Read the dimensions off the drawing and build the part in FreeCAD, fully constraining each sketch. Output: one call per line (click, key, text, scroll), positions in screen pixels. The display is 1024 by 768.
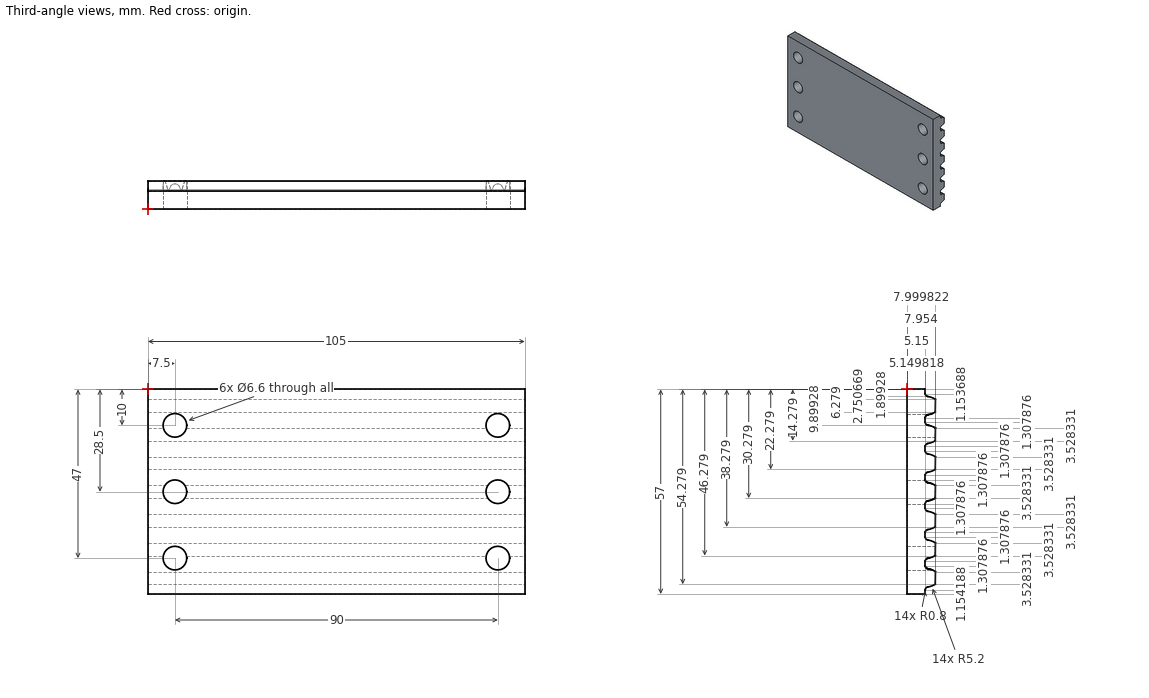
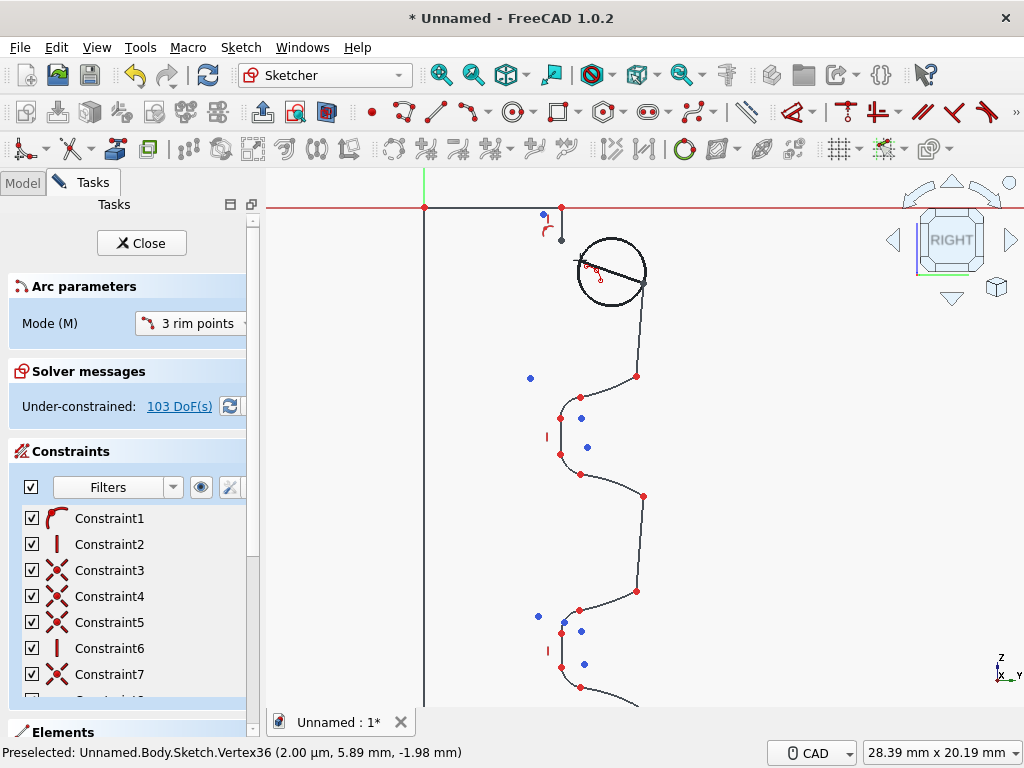
scroll(610, 267, up, 8)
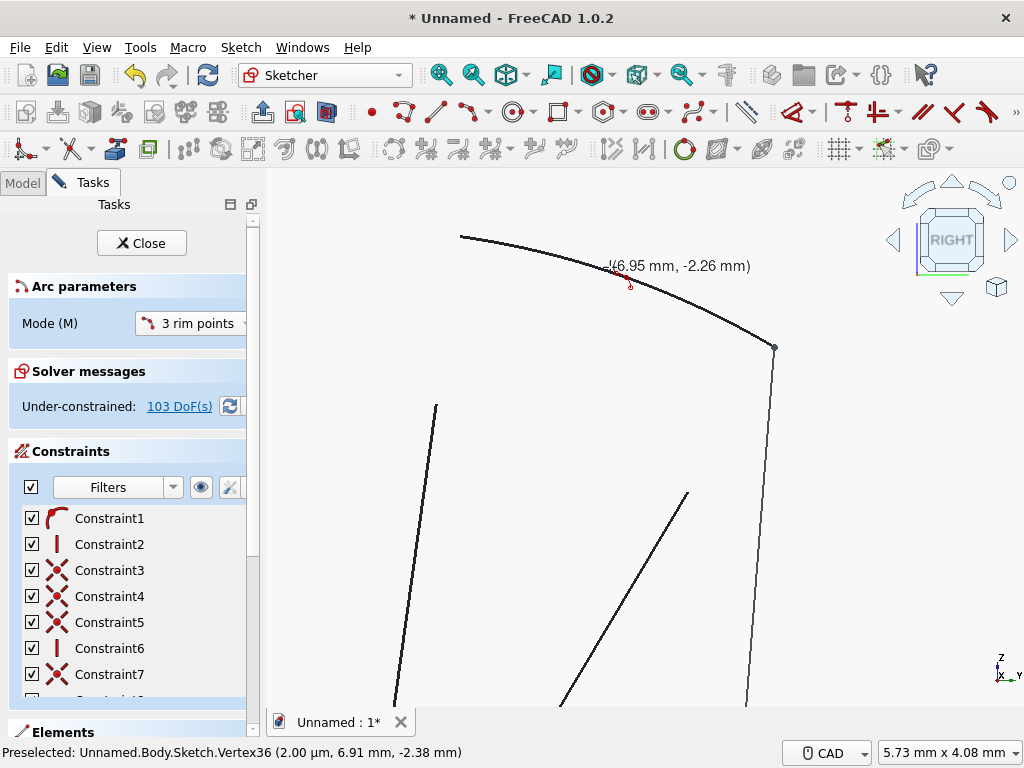
click(610, 267)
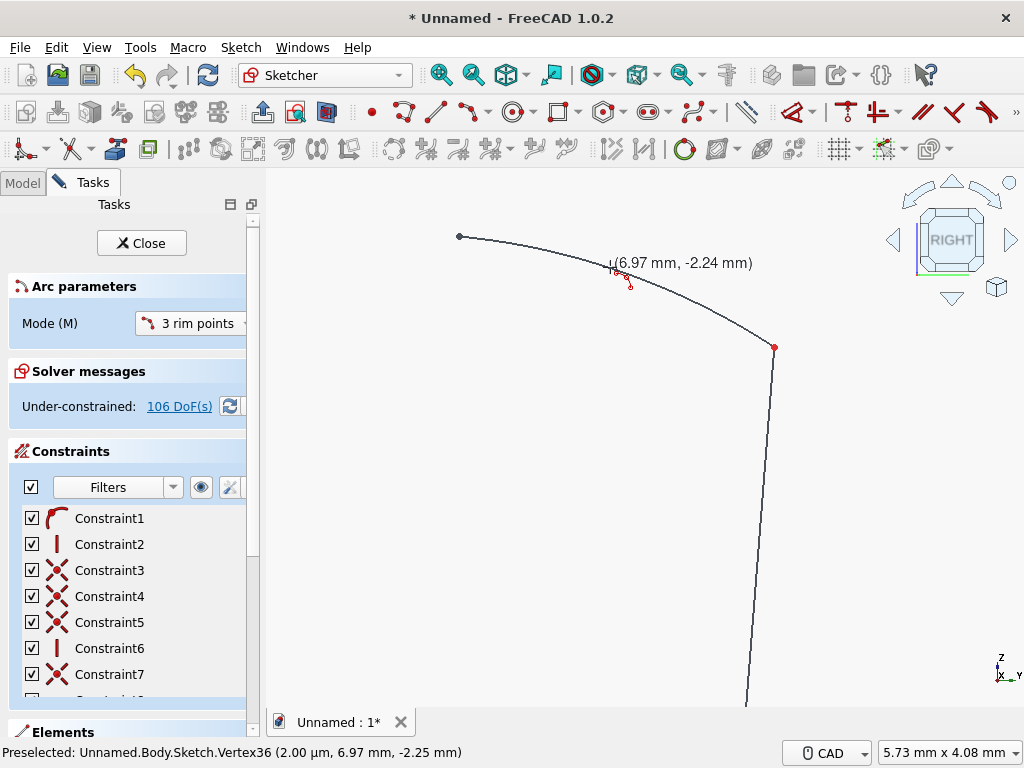
scroll(595, 264, down, 15)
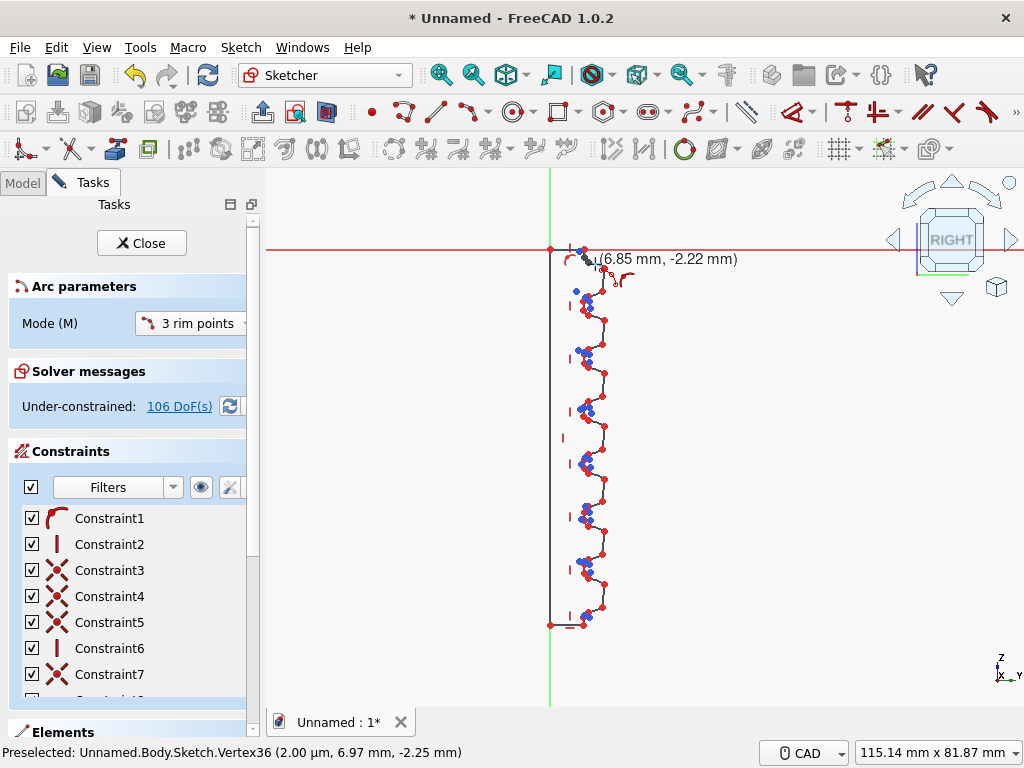
scroll(589, 262, up, 7)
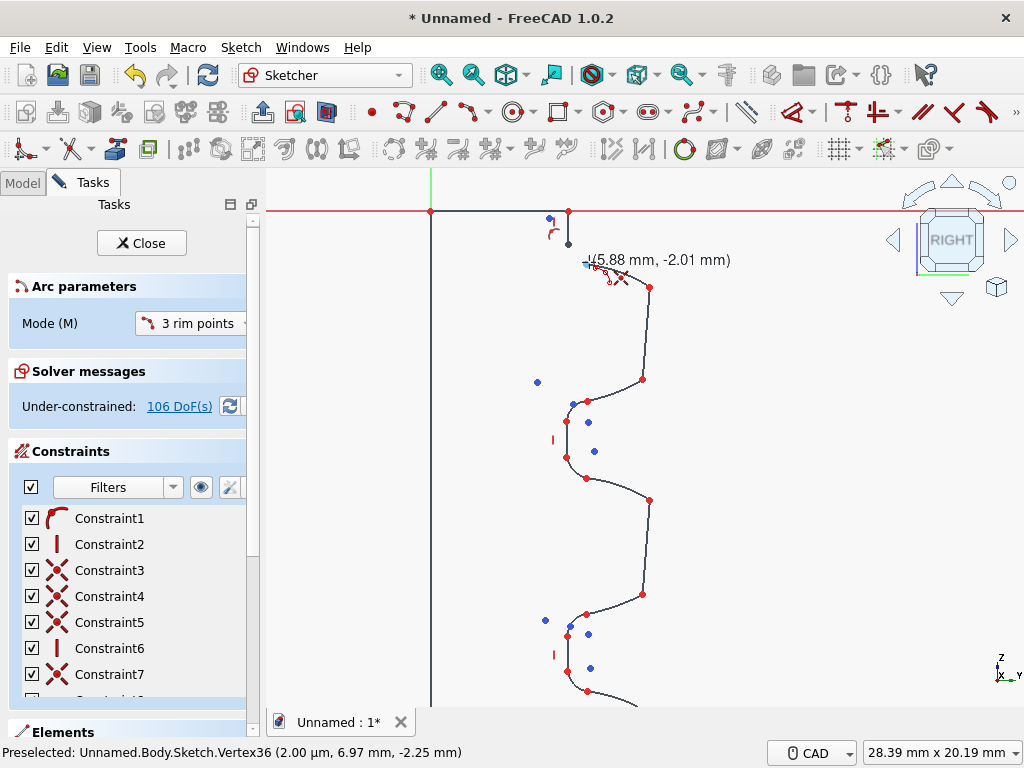
click(586, 265)
click(568, 244)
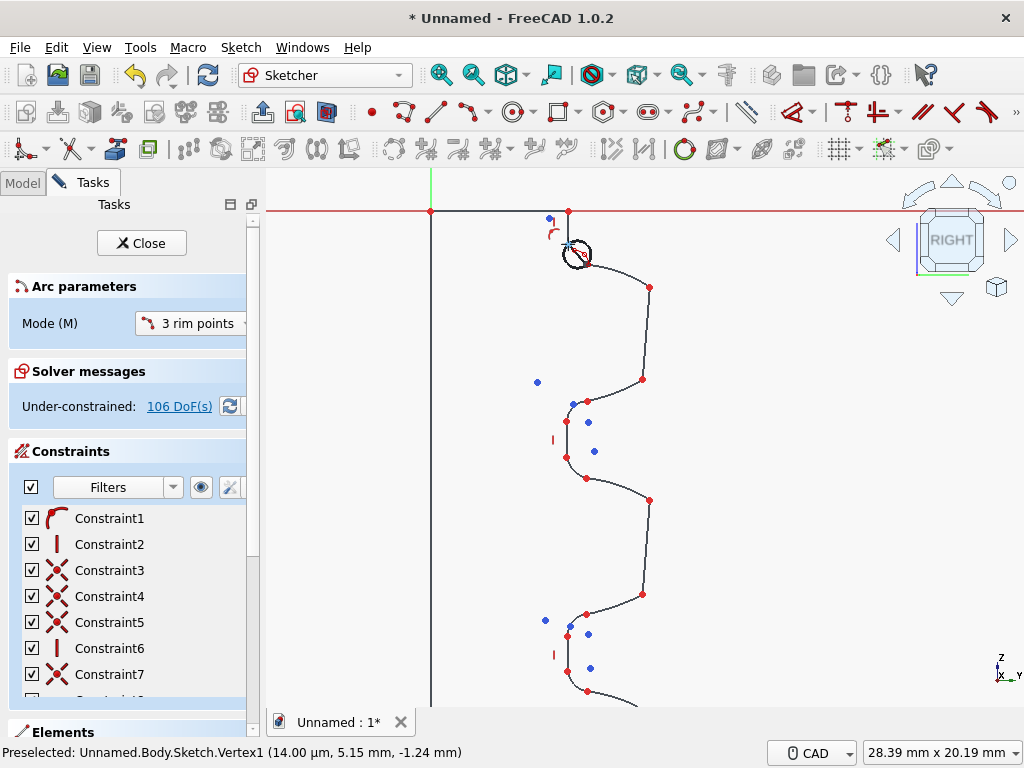
scroll(573, 256, up, 6)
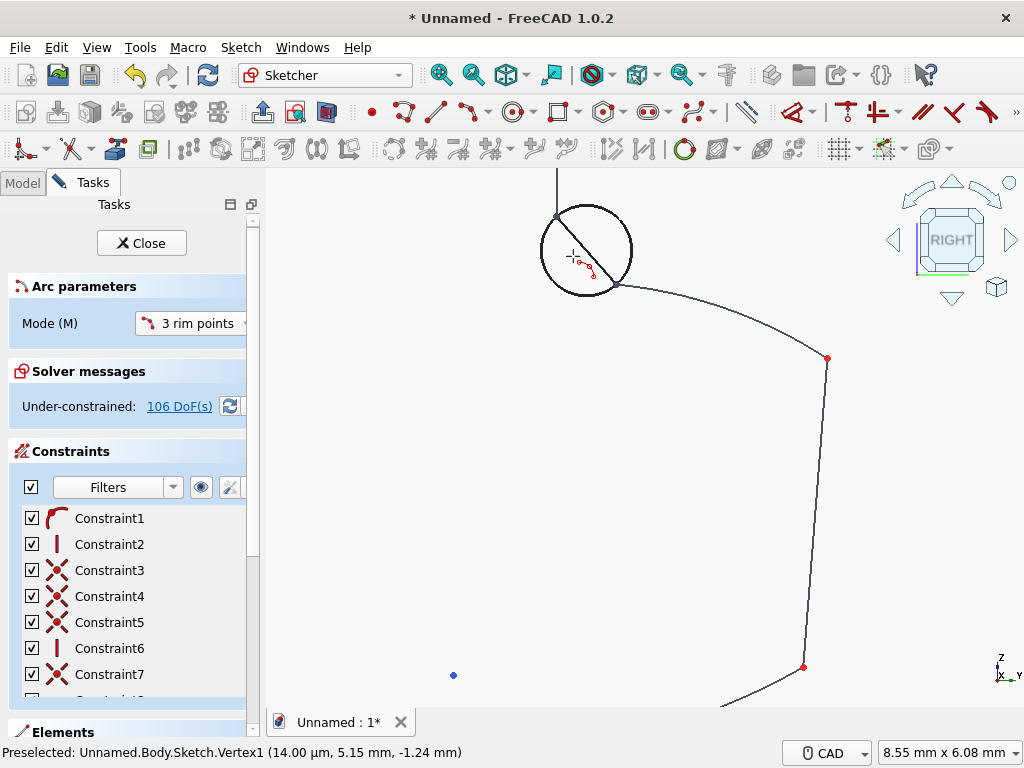
click(574, 256)
key(Escape)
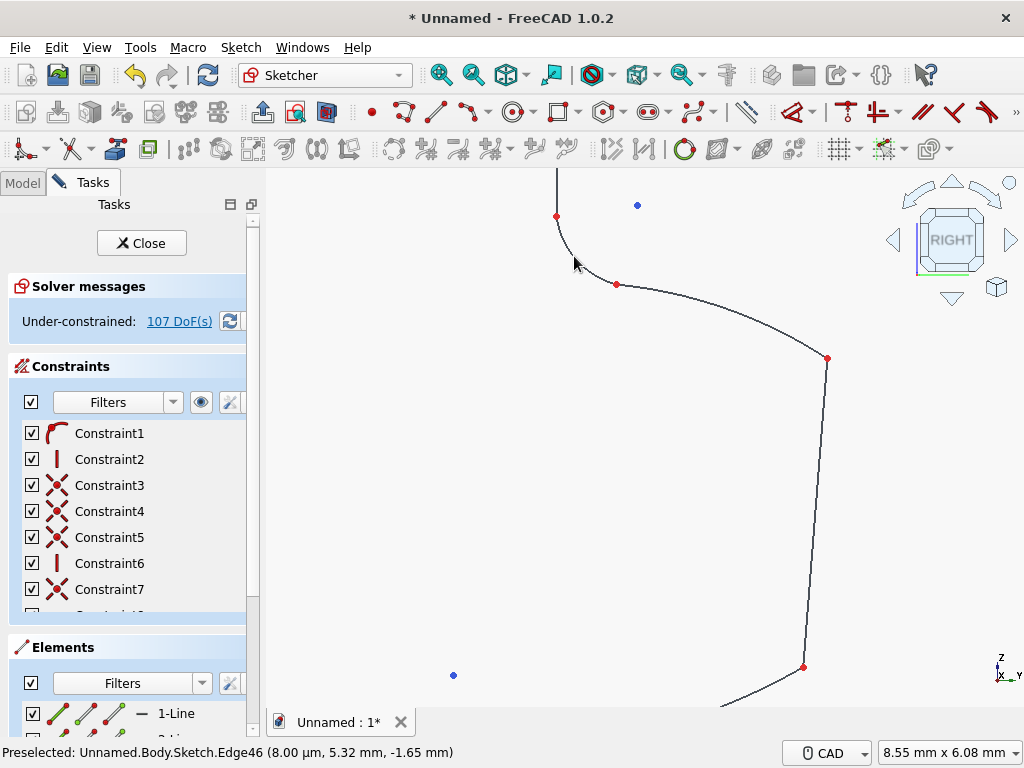
scroll(586, 261, down, 13)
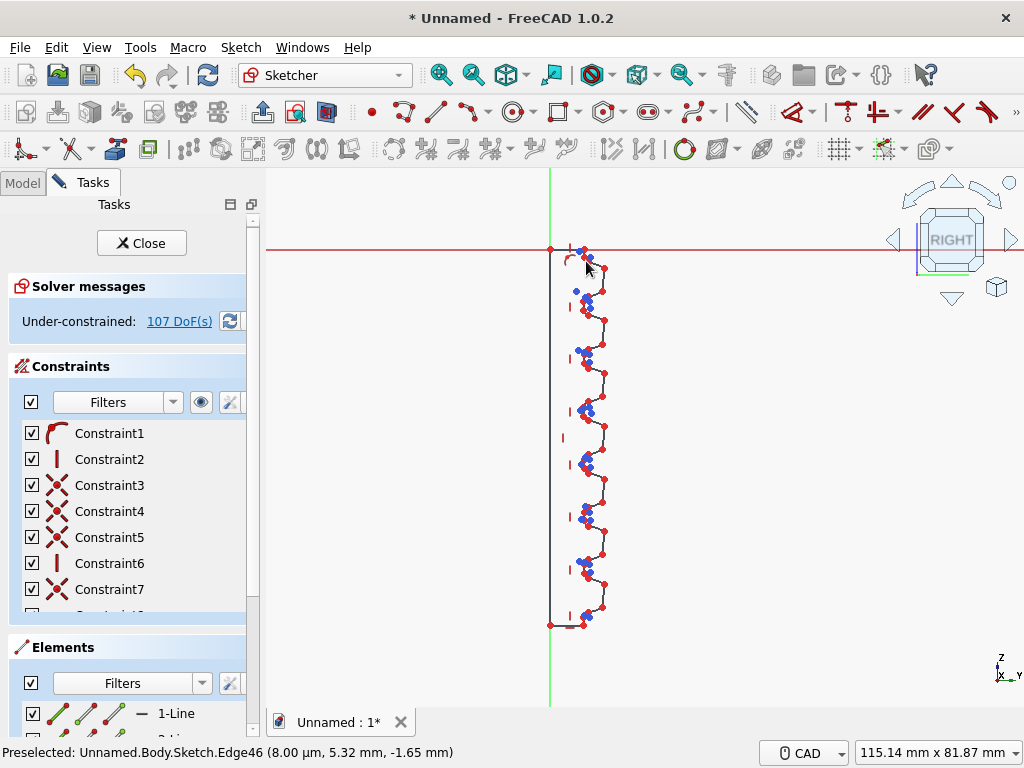
scroll(584, 255, up, 9)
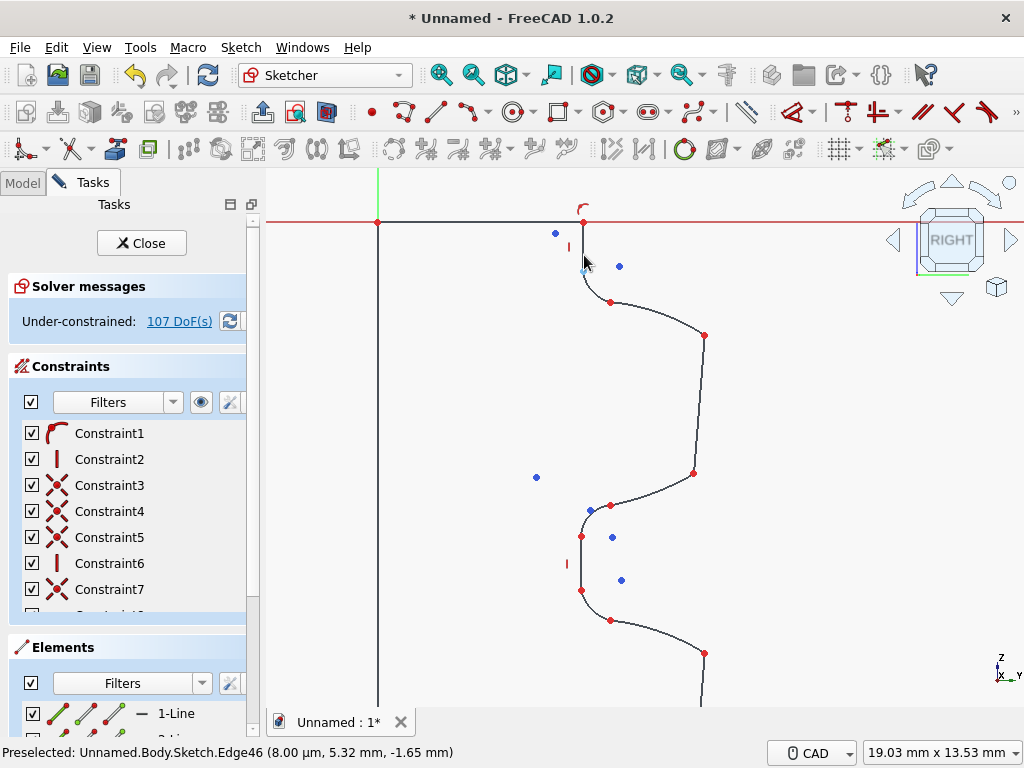
click(583, 257)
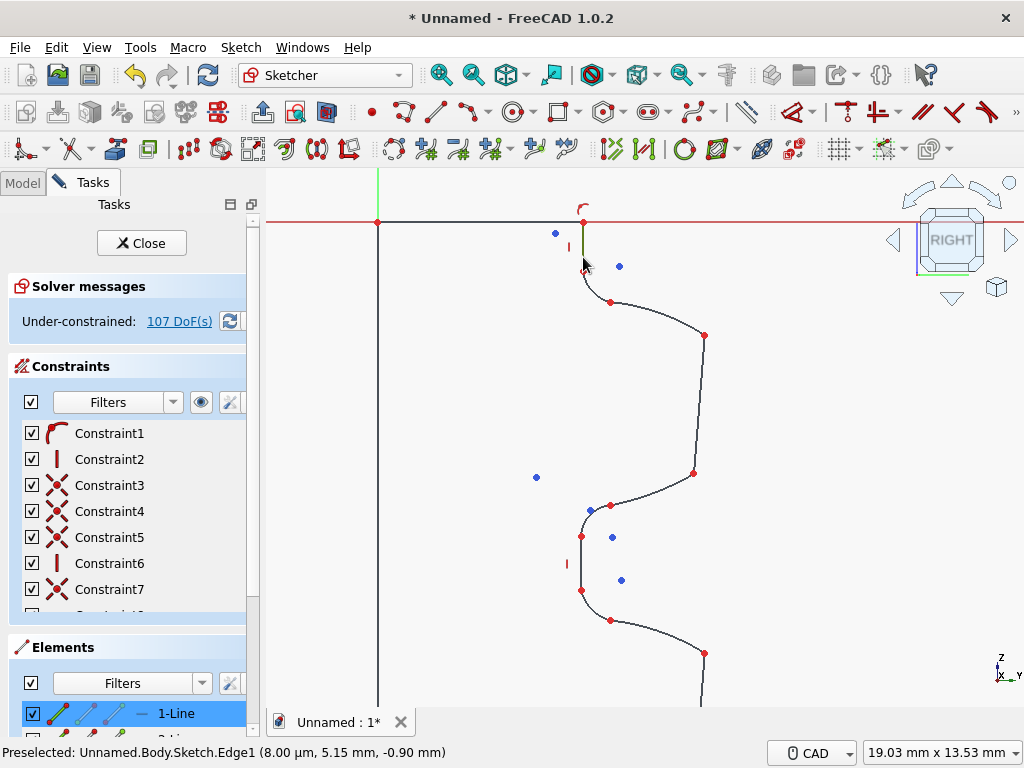
click(587, 284)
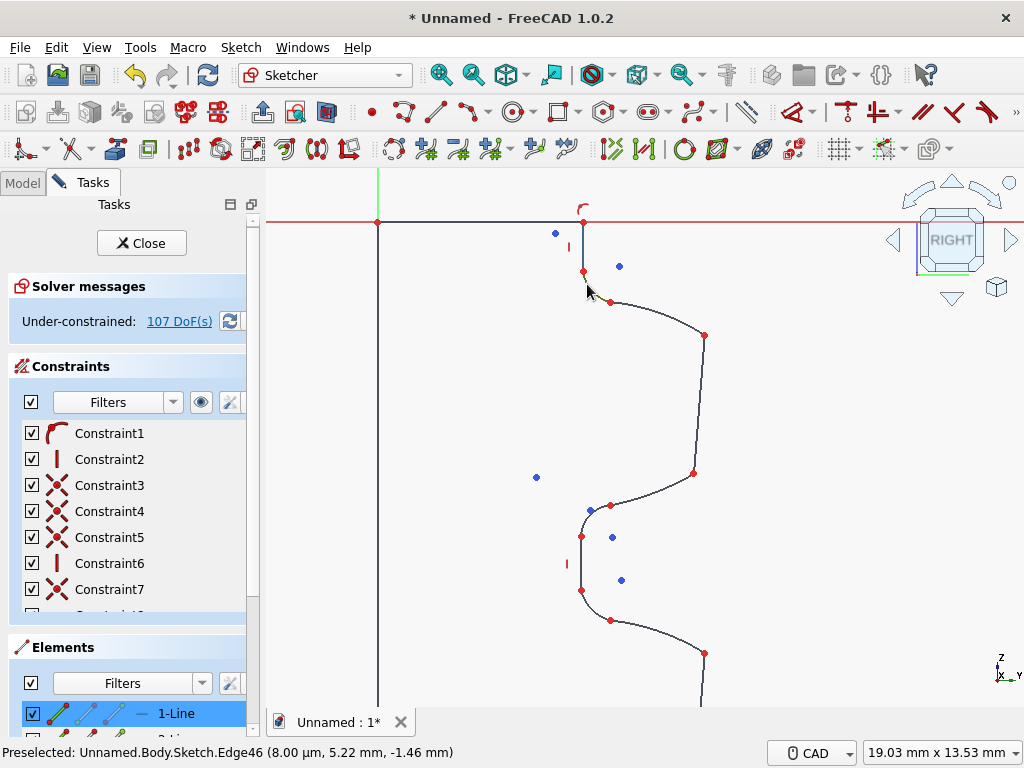
click(988, 112)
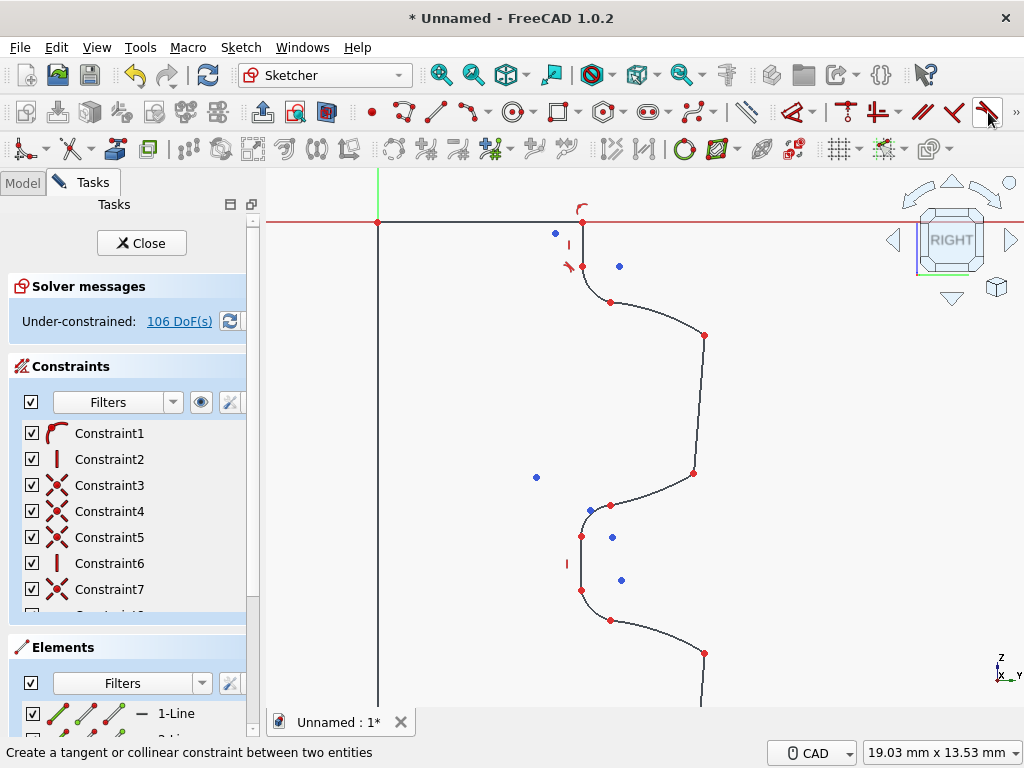
scroll(584, 255, down, 9)